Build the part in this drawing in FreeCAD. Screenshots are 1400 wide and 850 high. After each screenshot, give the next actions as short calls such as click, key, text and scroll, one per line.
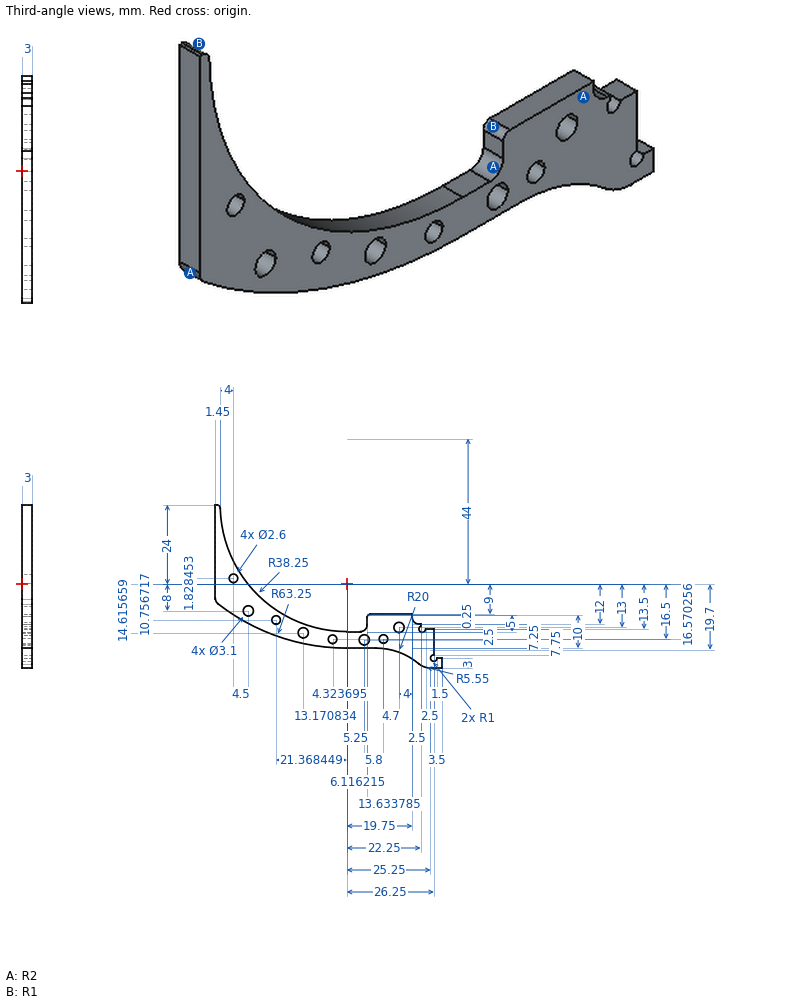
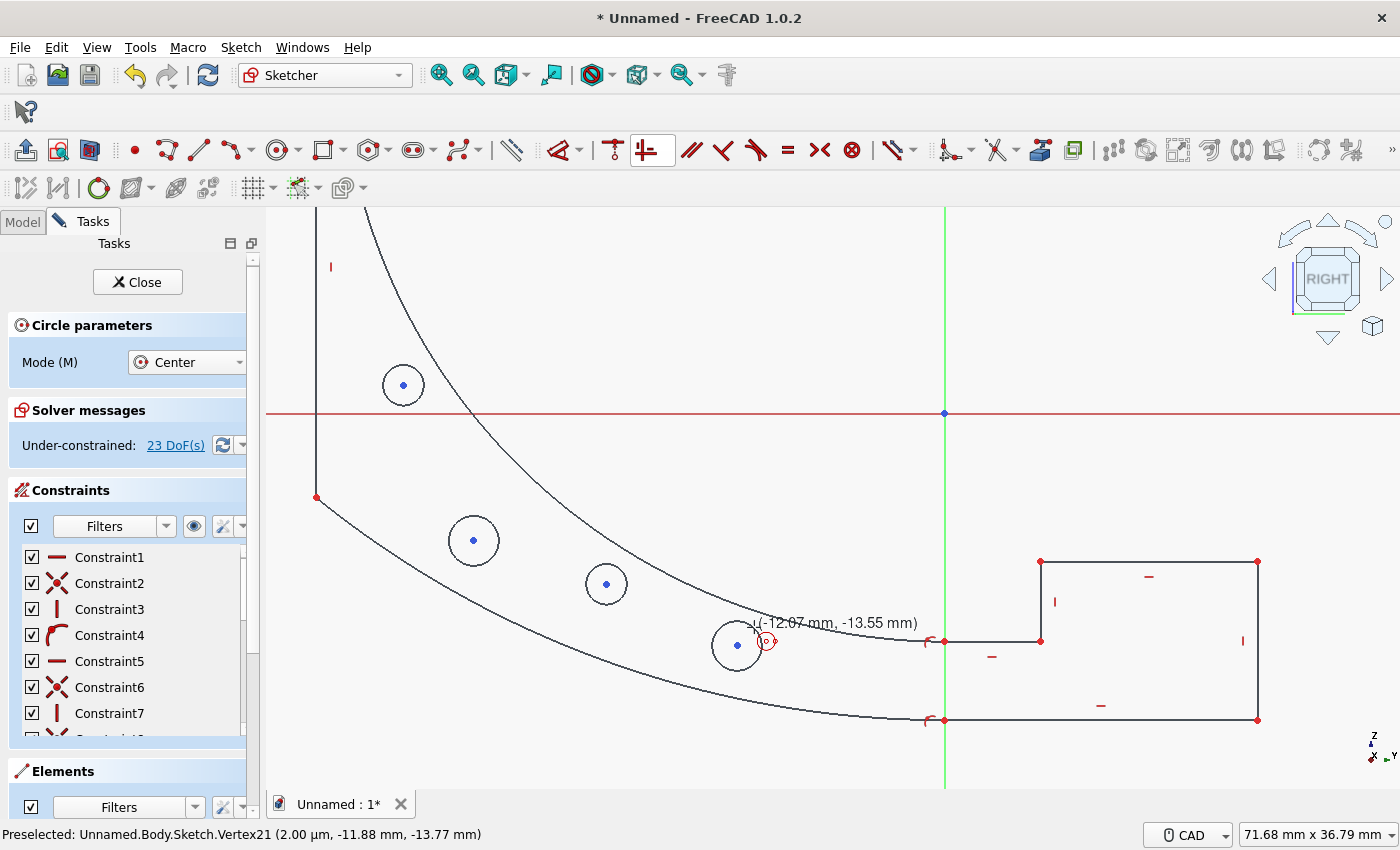
click(877, 676)
click(891, 661)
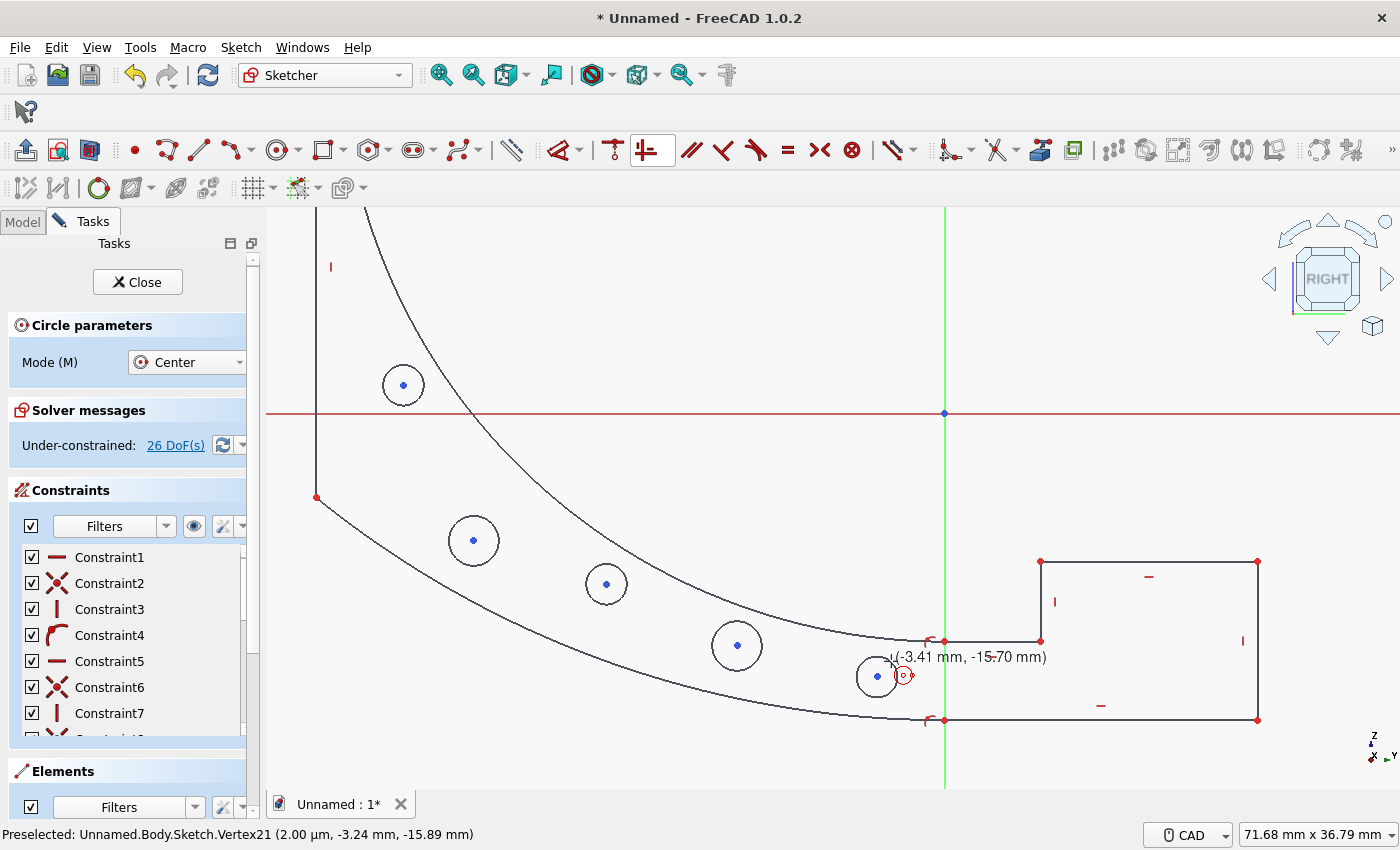
click(1028, 679)
click(1045, 661)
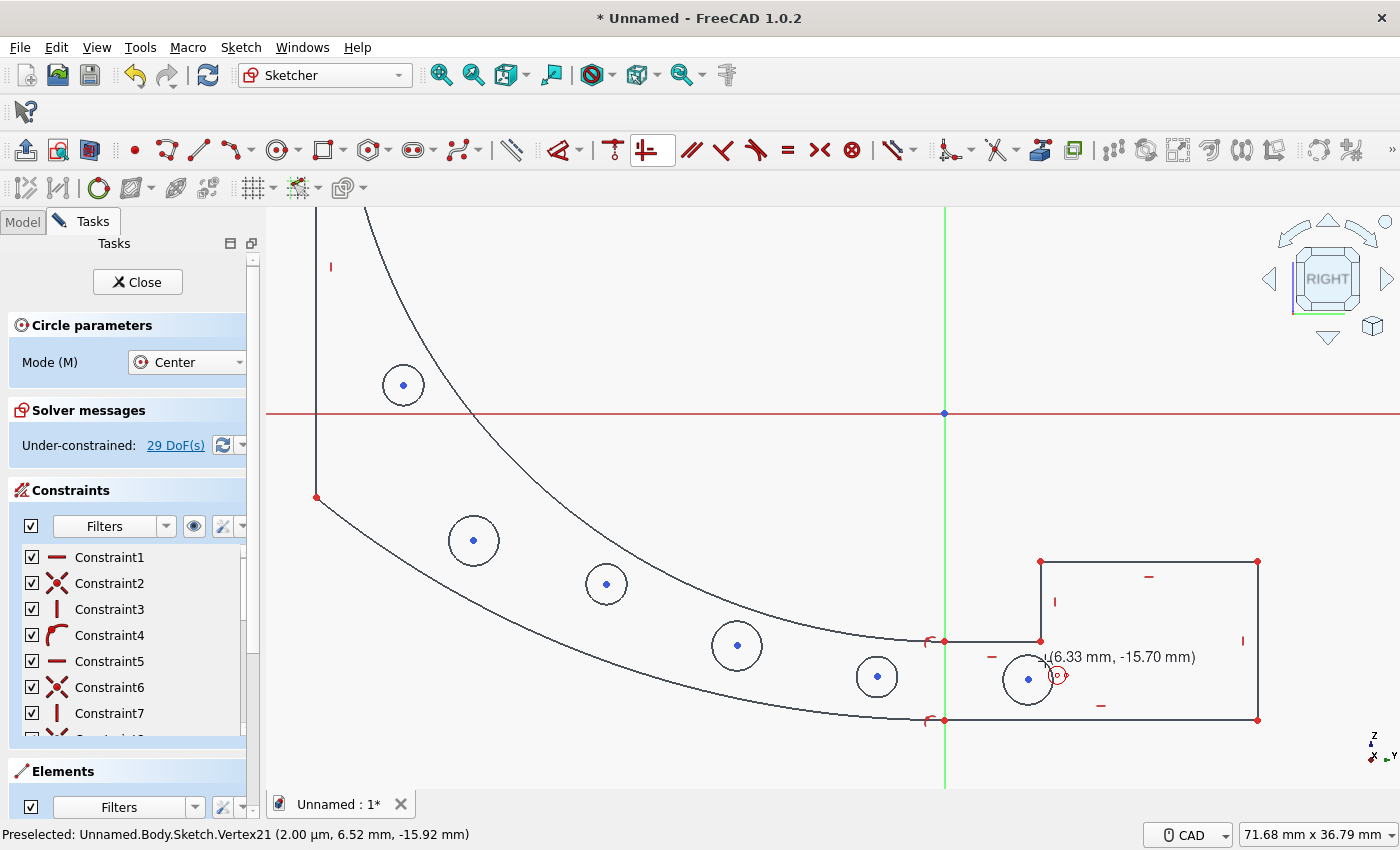
click(1194, 619)
click(1211, 602)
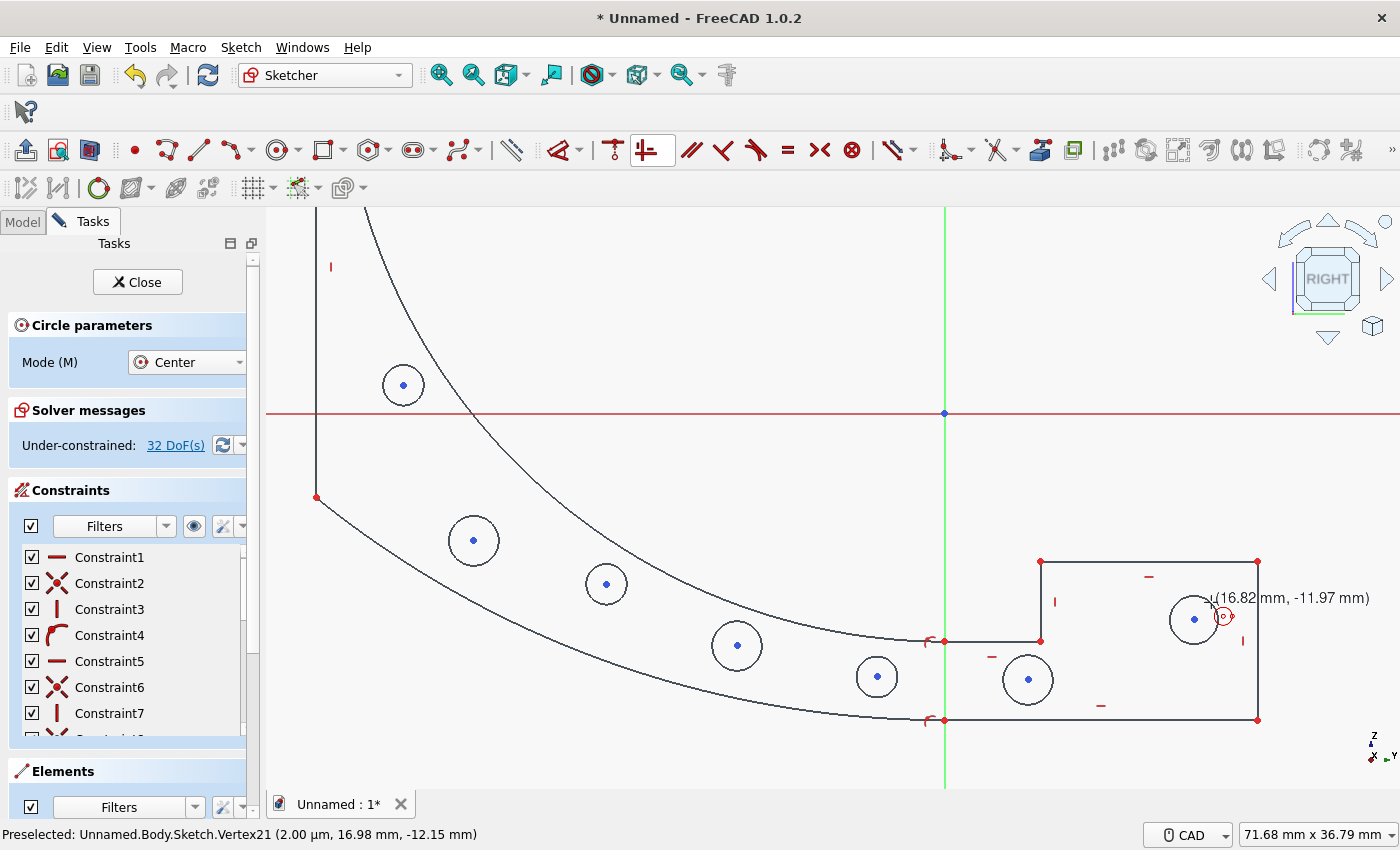
click(1120, 675)
click(1134, 660)
key(Escape)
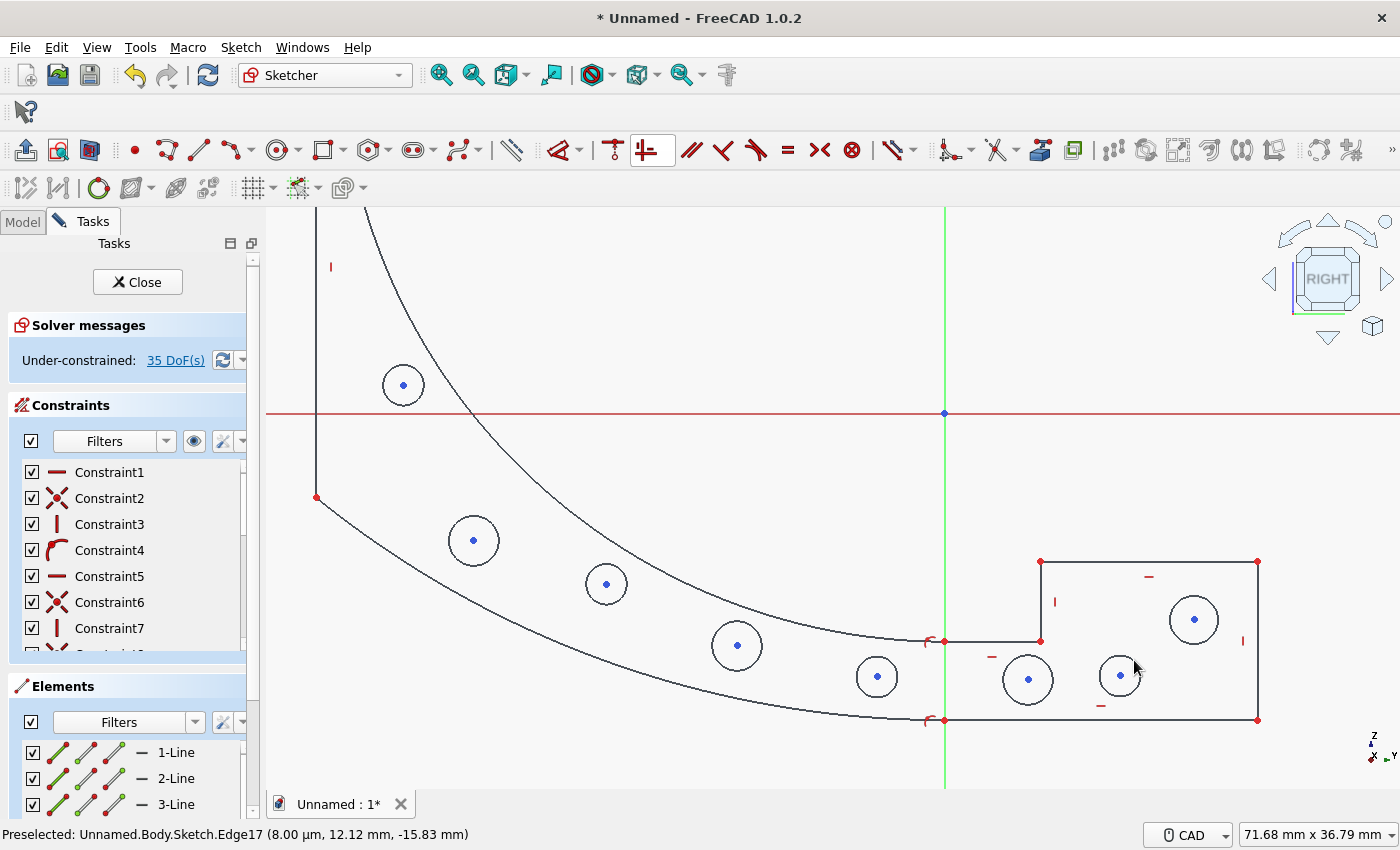
click(418, 371)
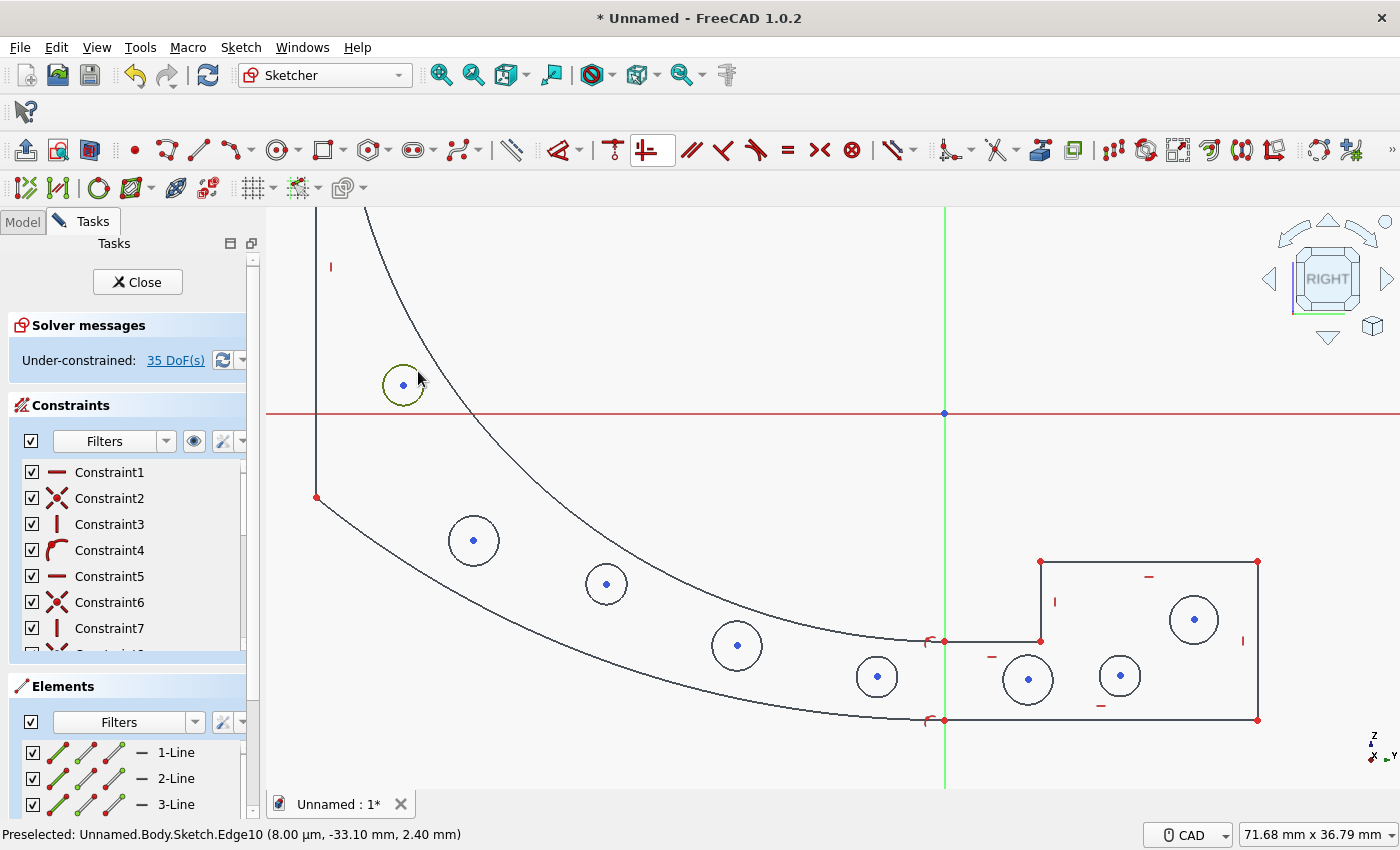
click(621, 570)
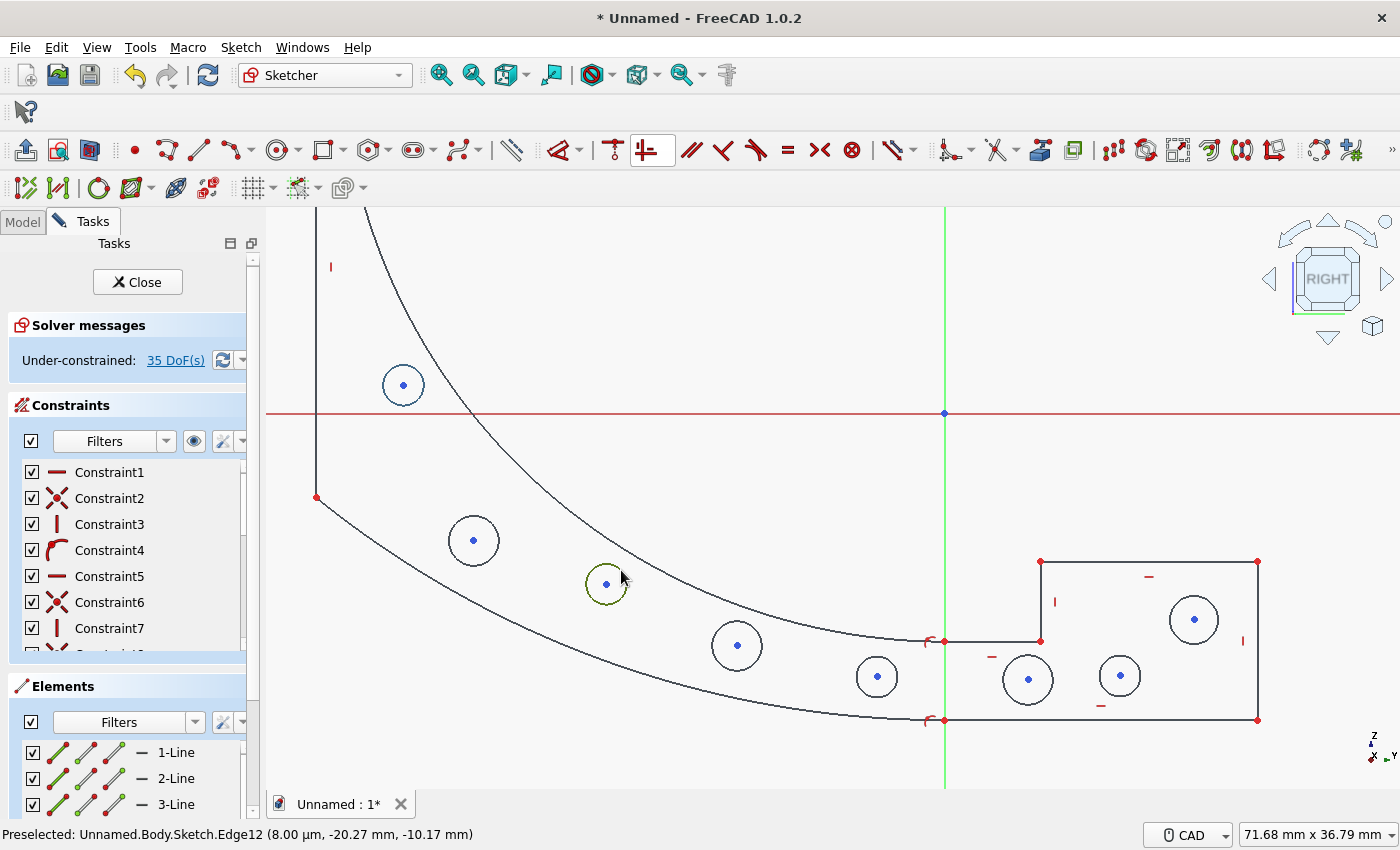
click(891, 662)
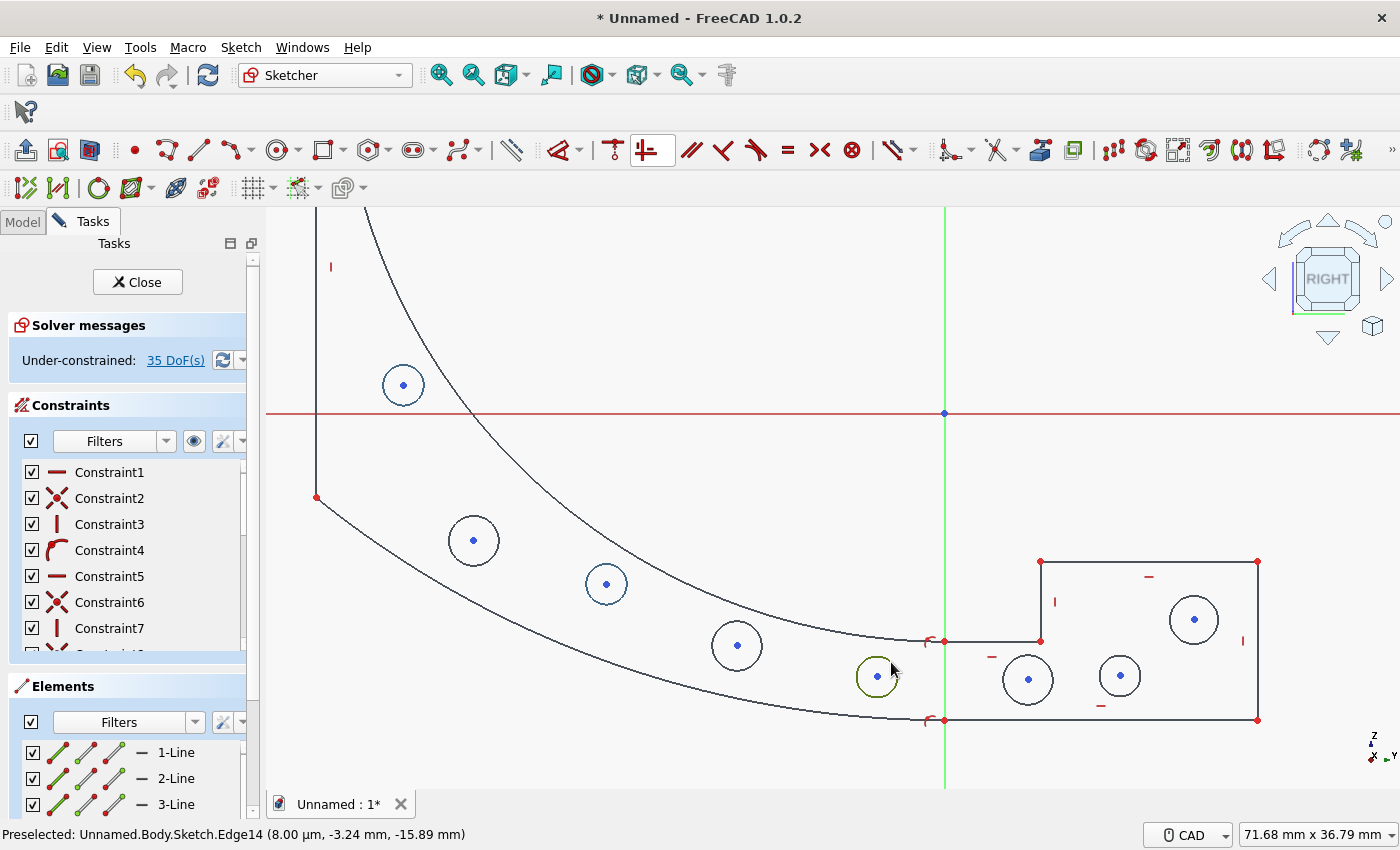
click(1134, 661)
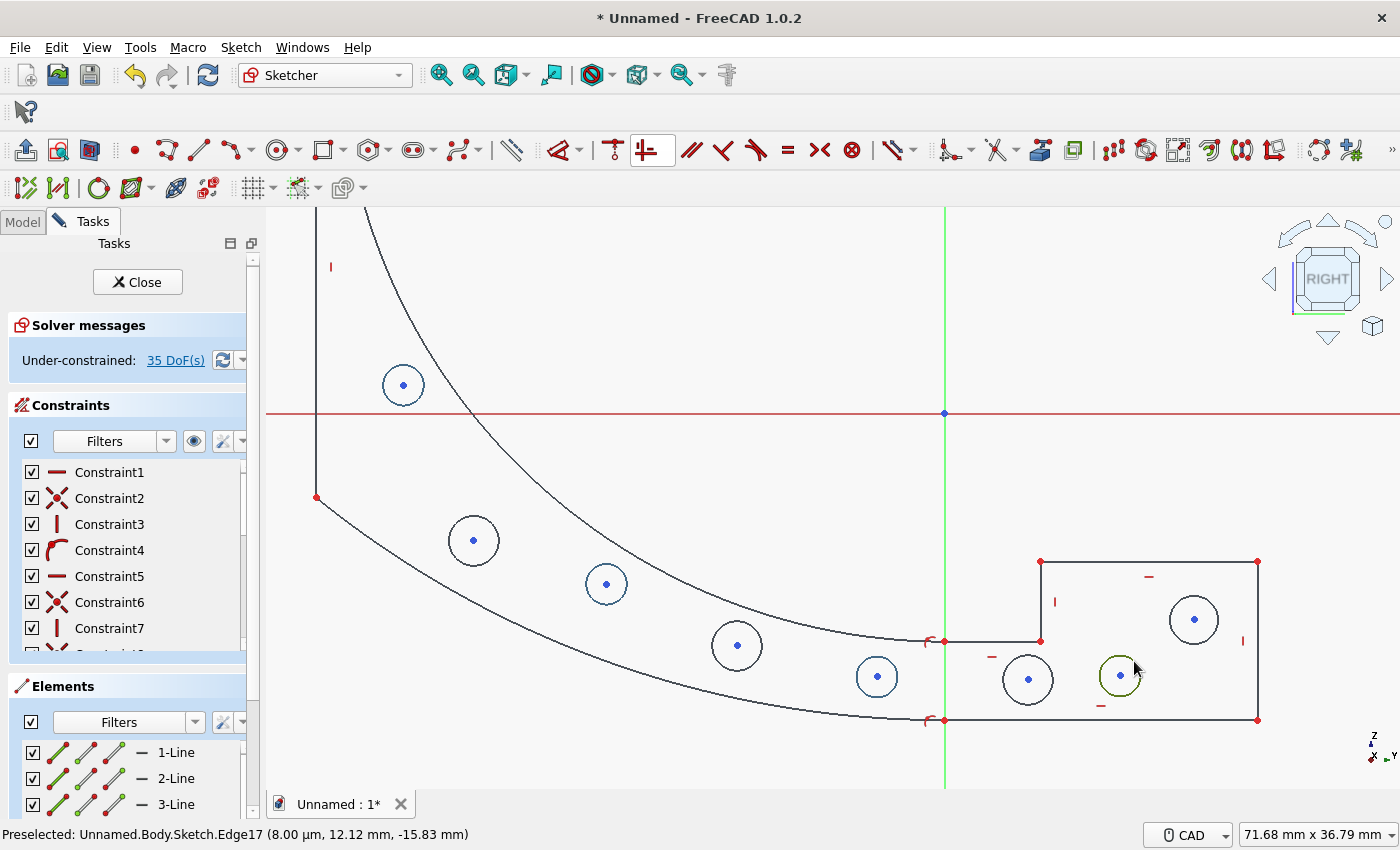
key(e)